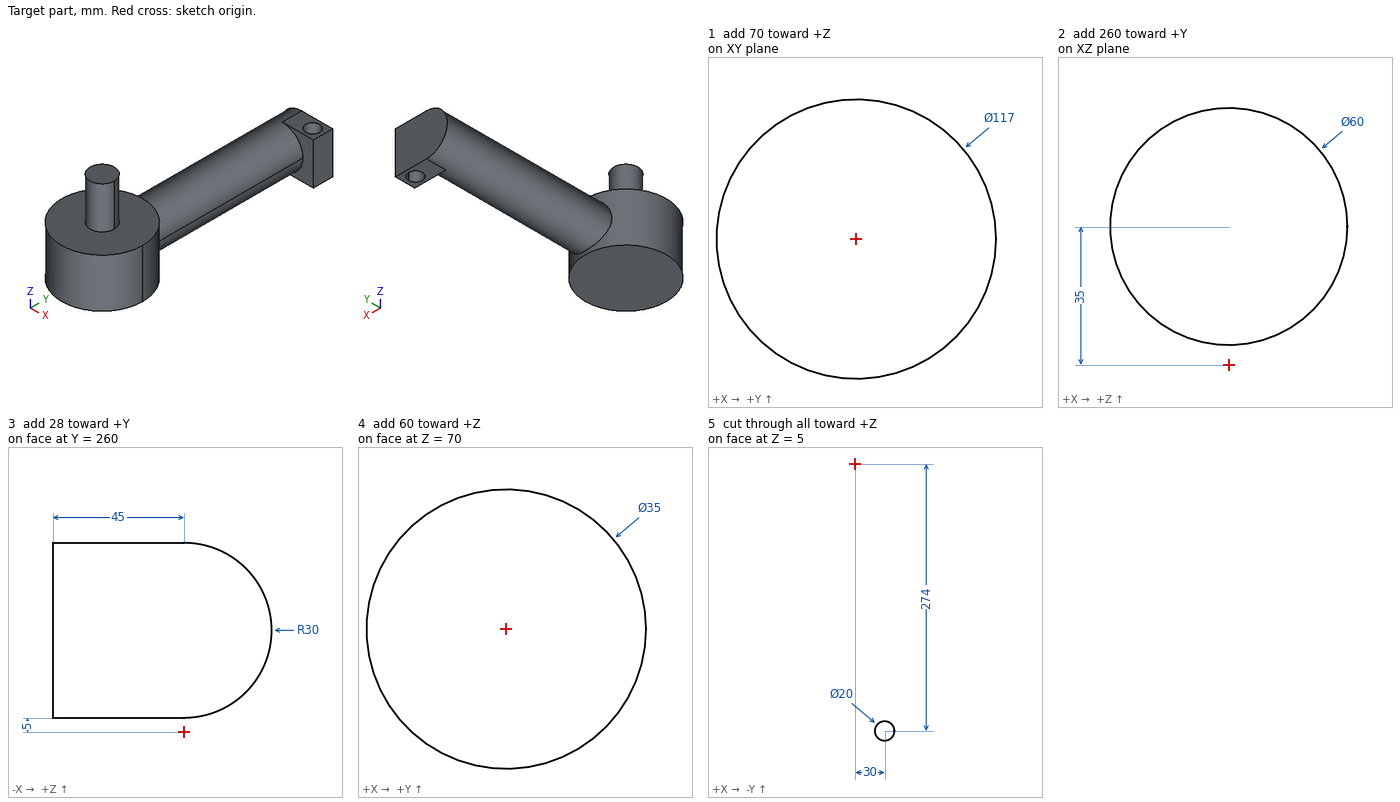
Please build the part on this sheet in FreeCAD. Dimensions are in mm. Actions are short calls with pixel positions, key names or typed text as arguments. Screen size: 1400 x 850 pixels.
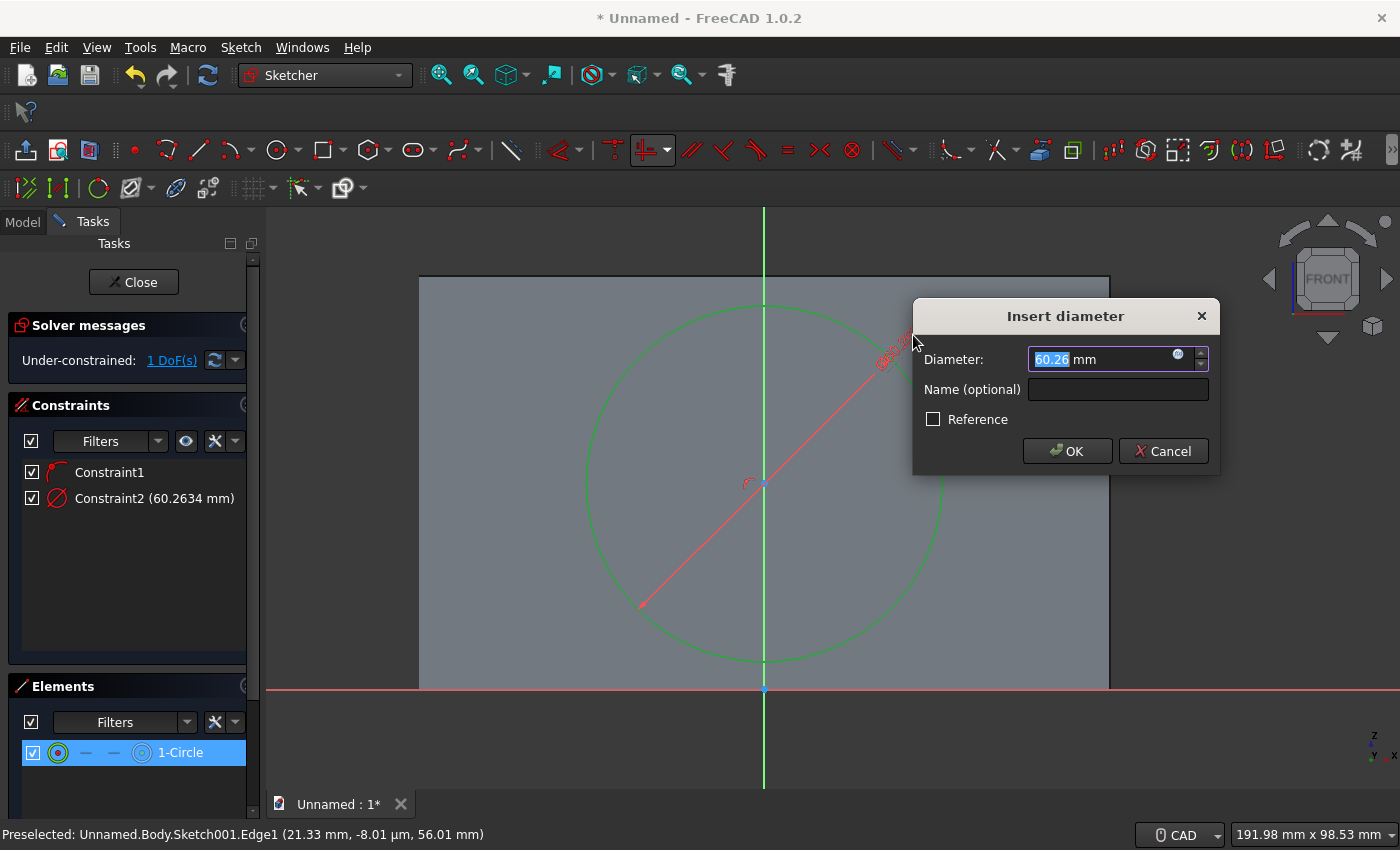
text(60)
key(Return)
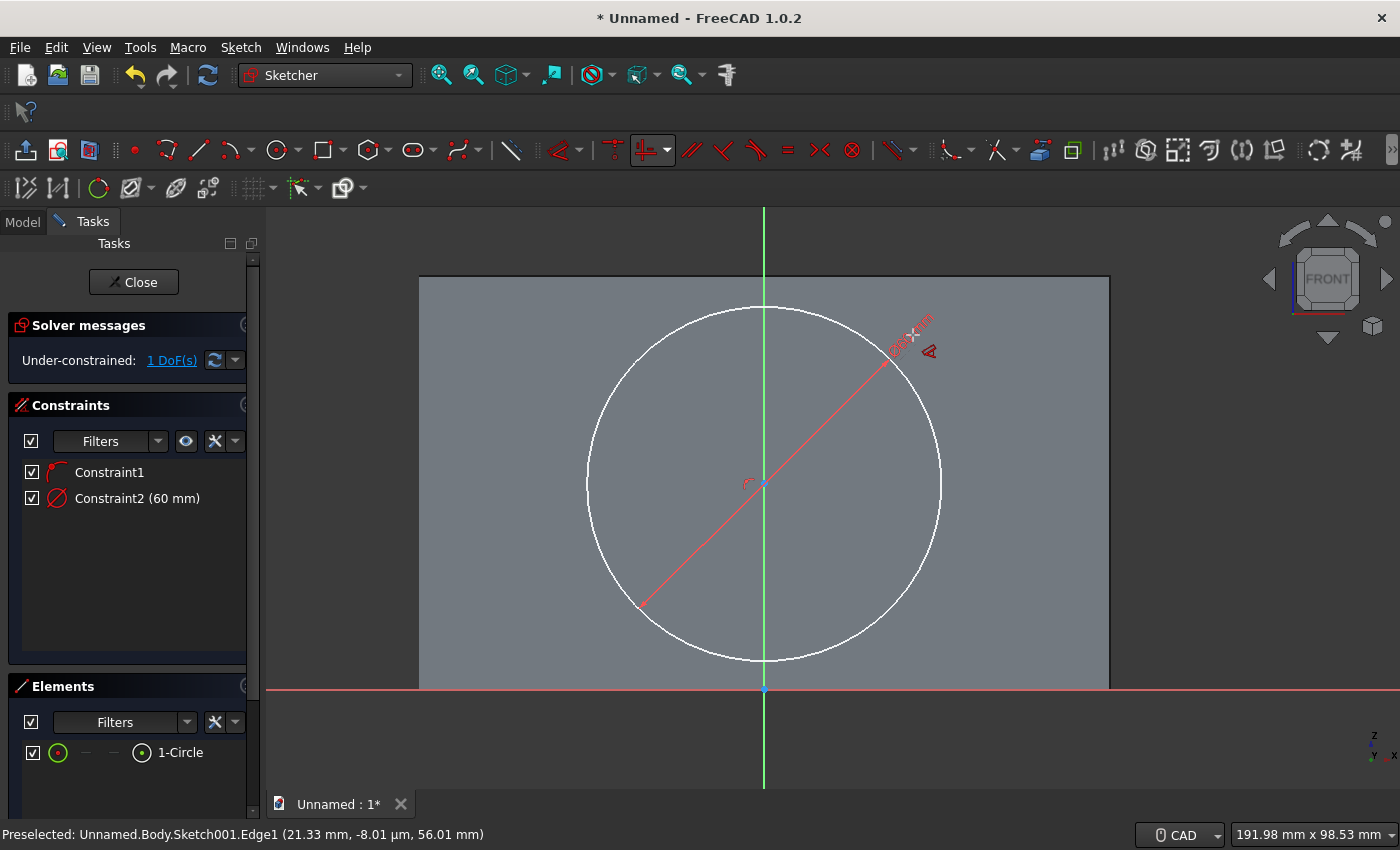
click(764, 484)
click(798, 587)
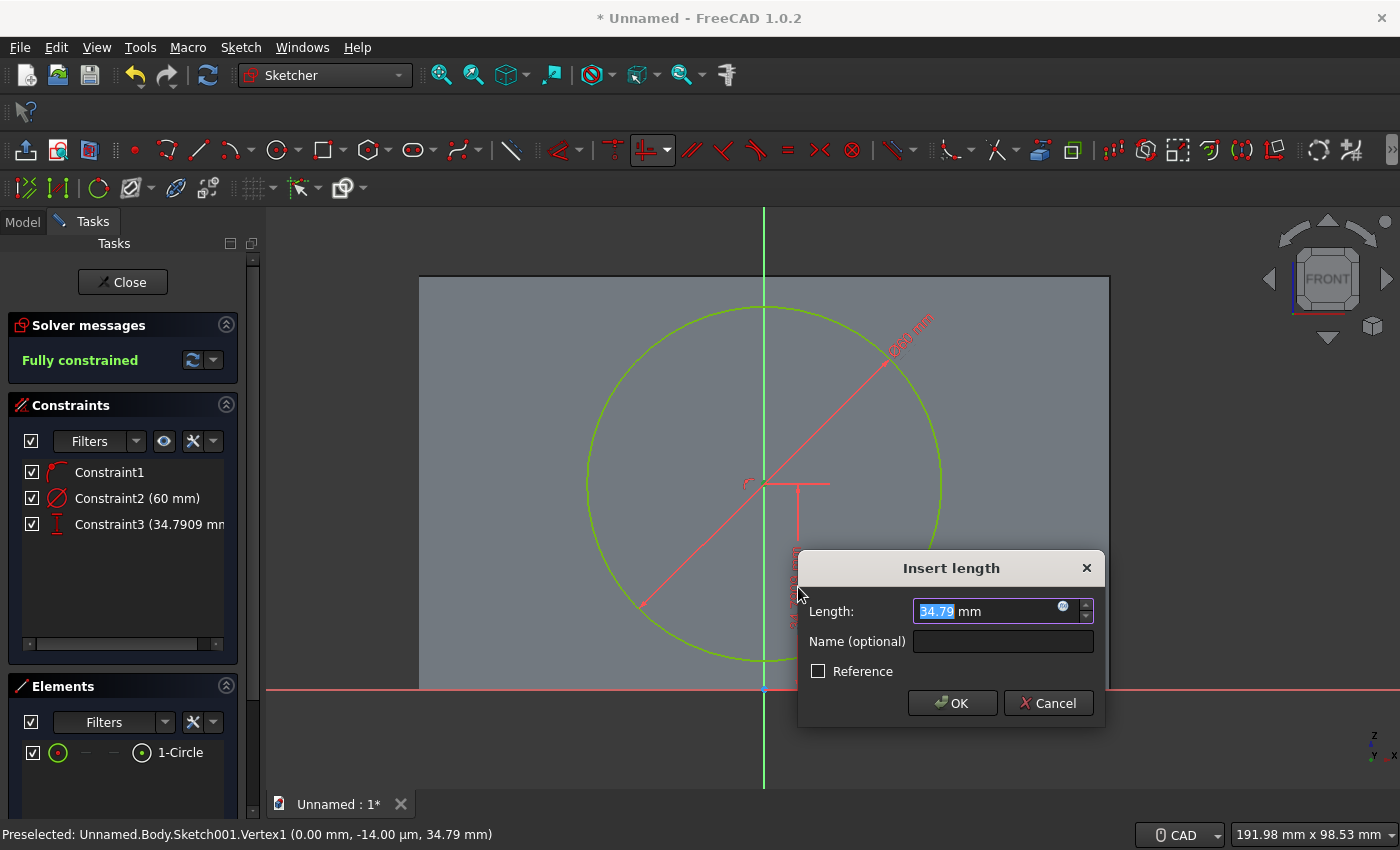
text(35)
key(Return)
key(Escape)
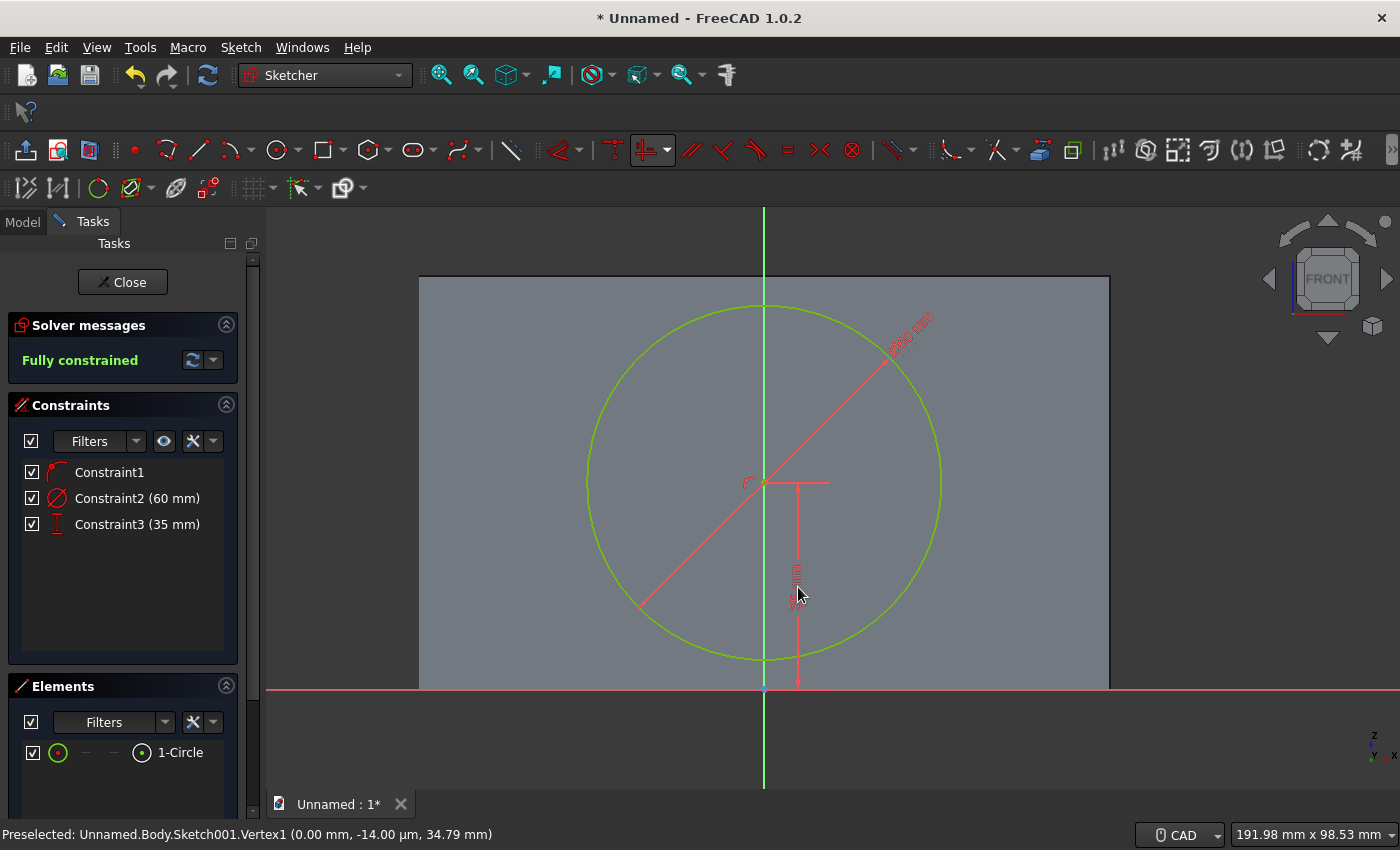
click(123, 282)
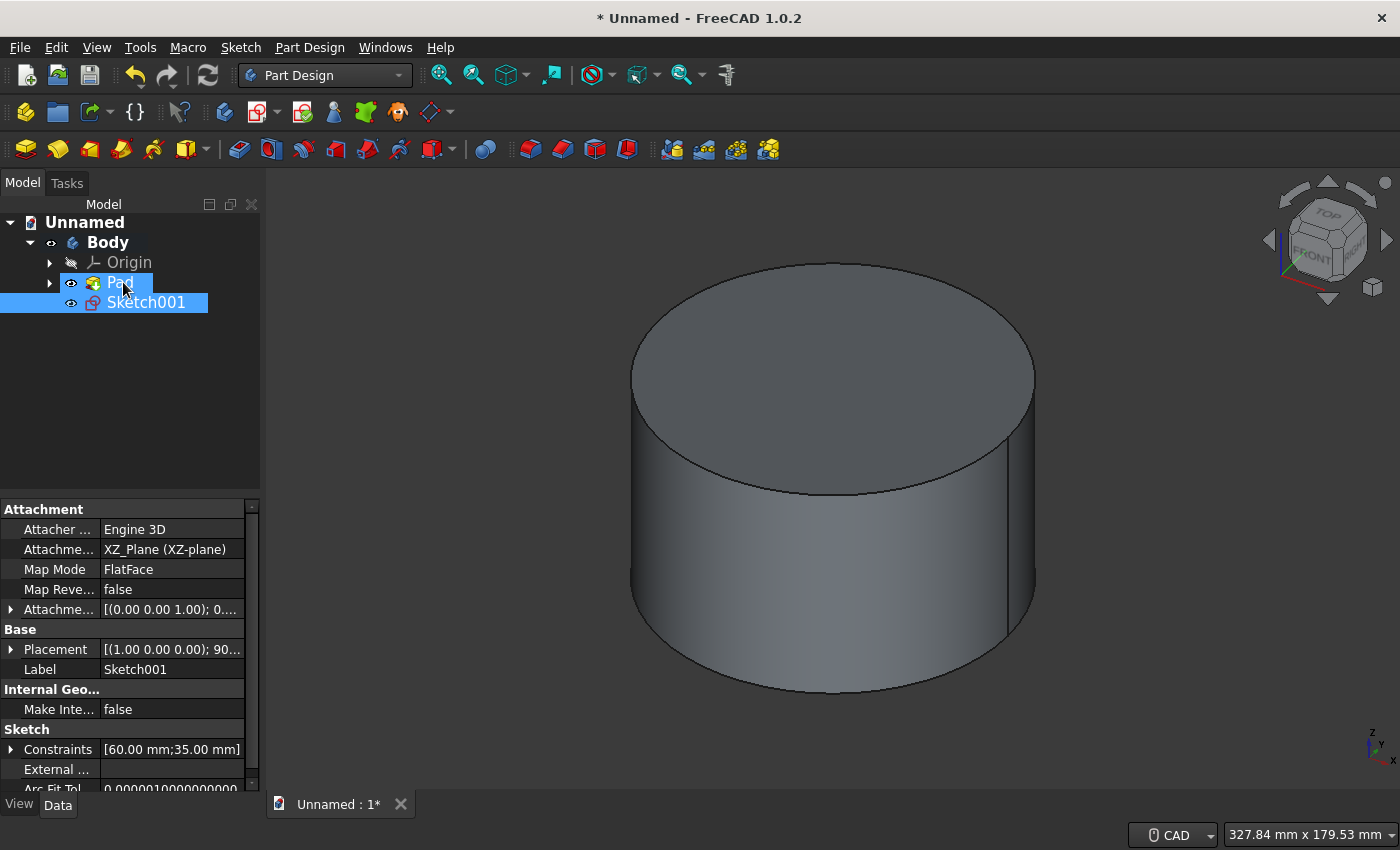
click(26, 150)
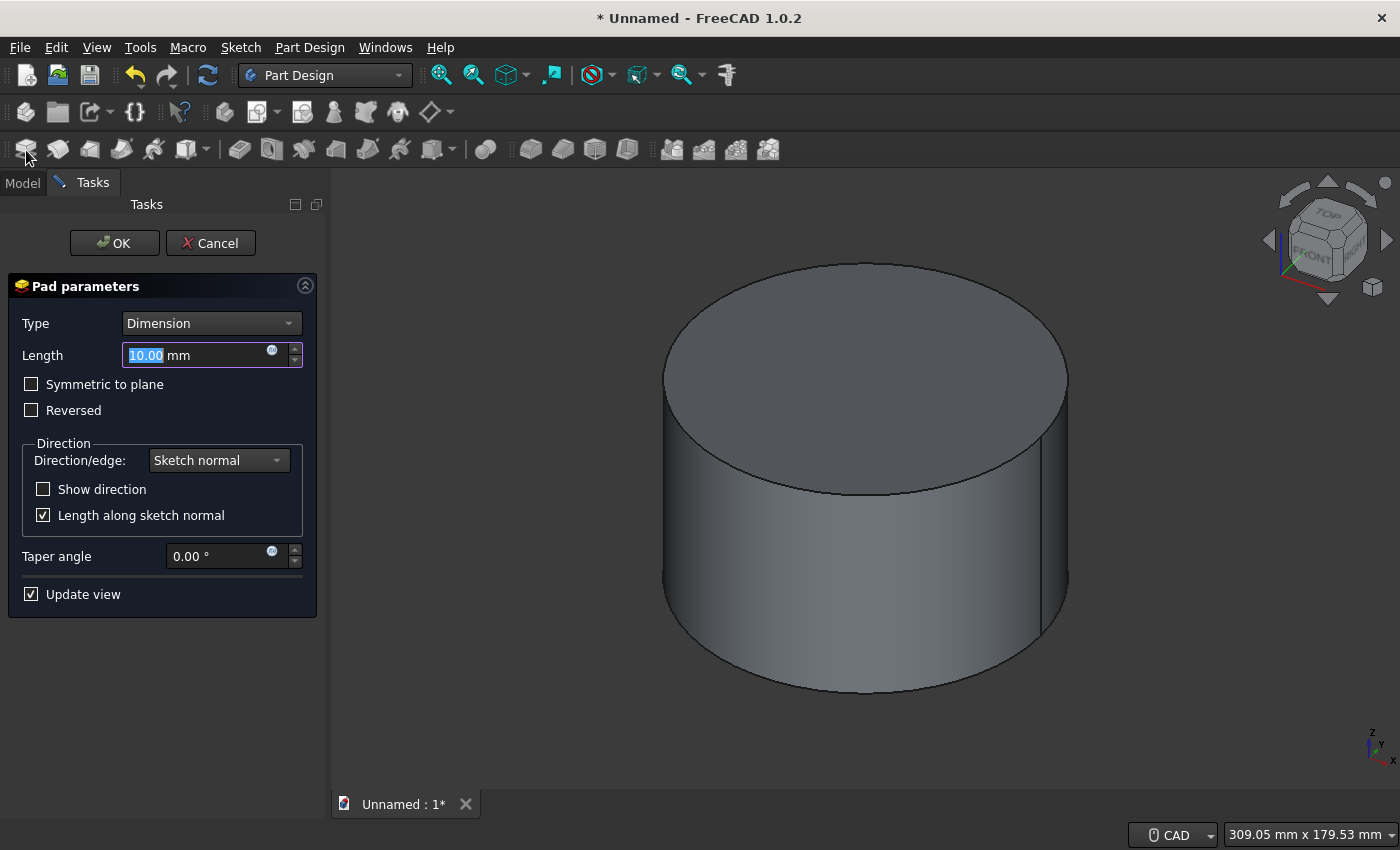
text(260)
key(Tab)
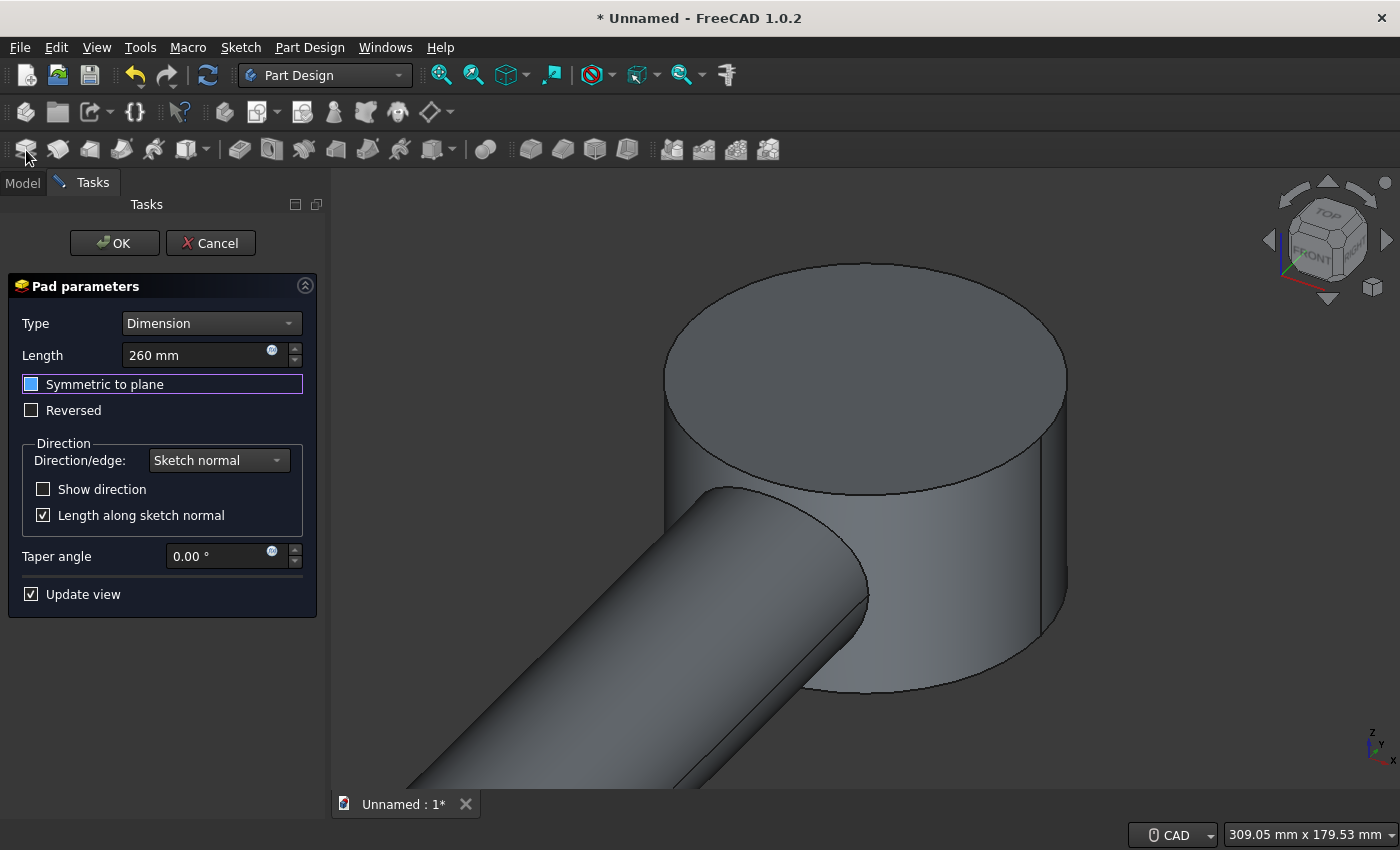
click(30, 410)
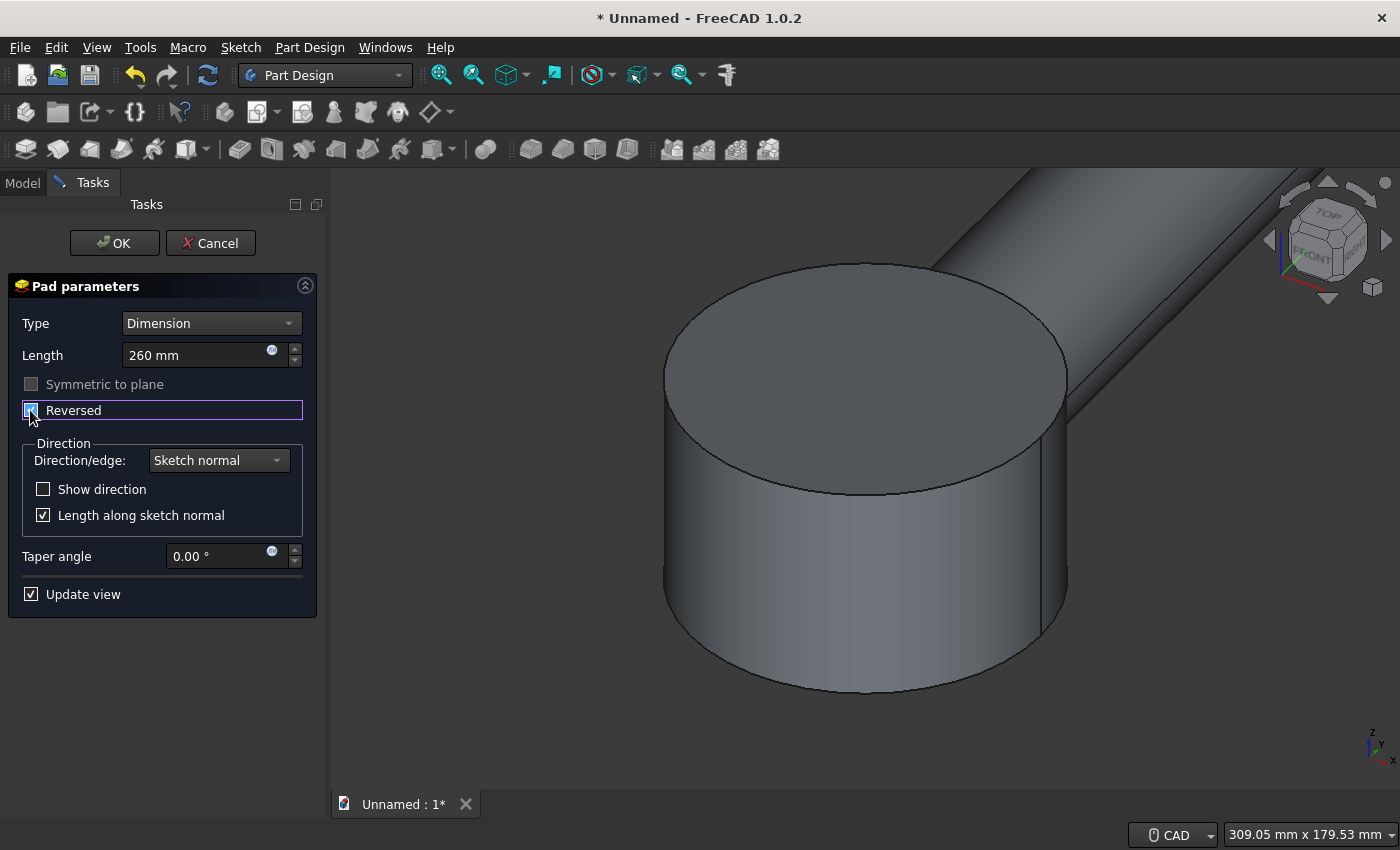
click(115, 243)